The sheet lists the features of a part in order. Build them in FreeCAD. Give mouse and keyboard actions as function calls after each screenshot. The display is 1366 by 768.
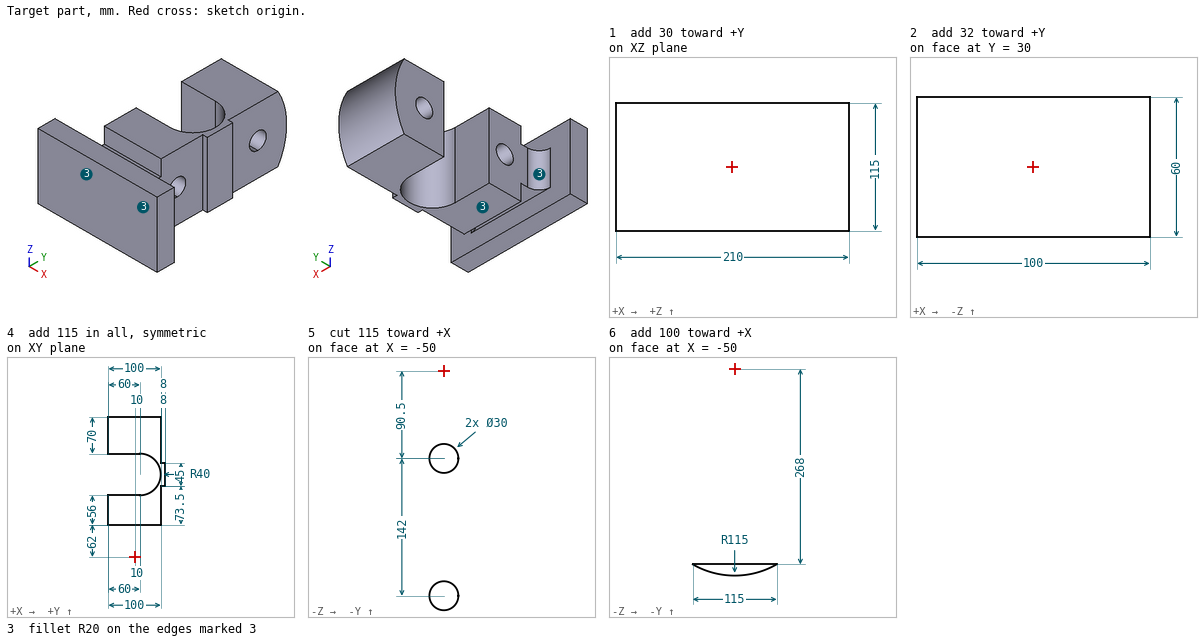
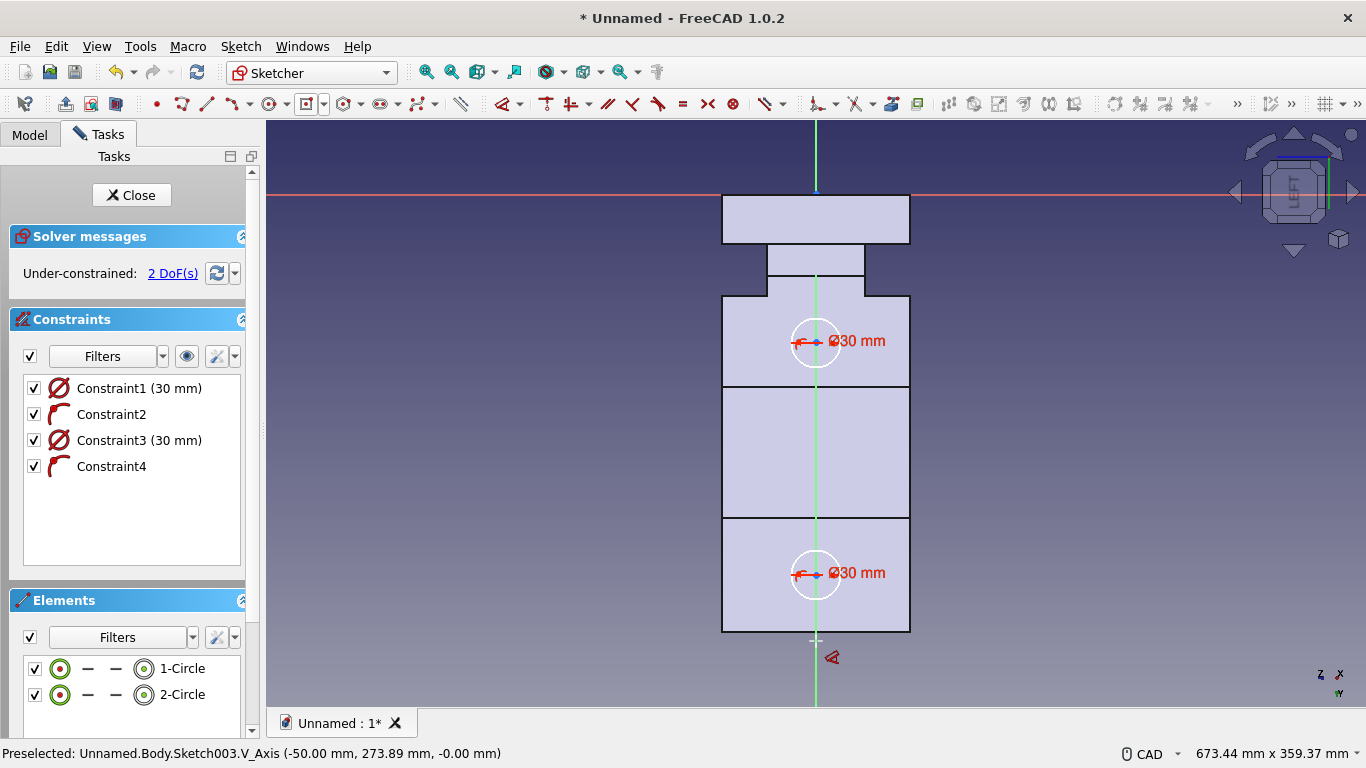
click(816, 343)
click(850, 269)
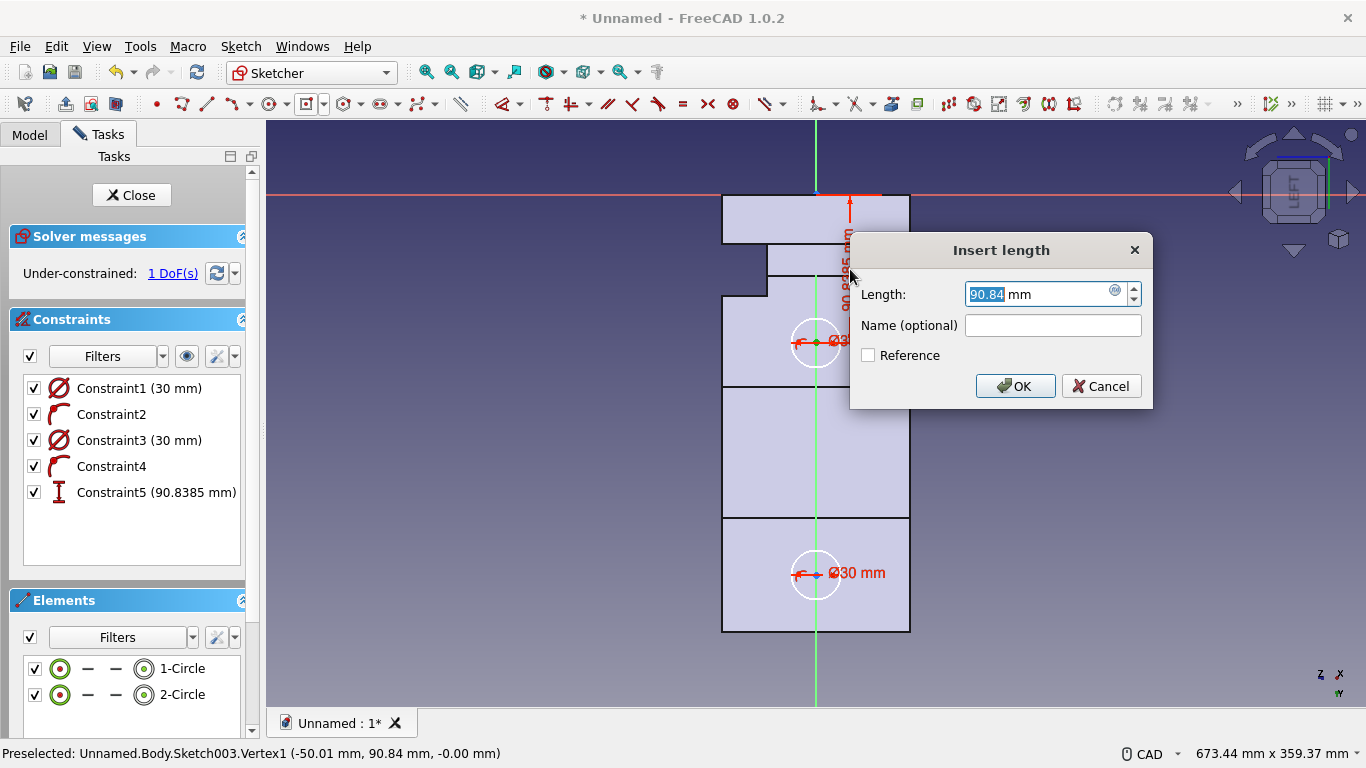
text(90.5)
key(Return)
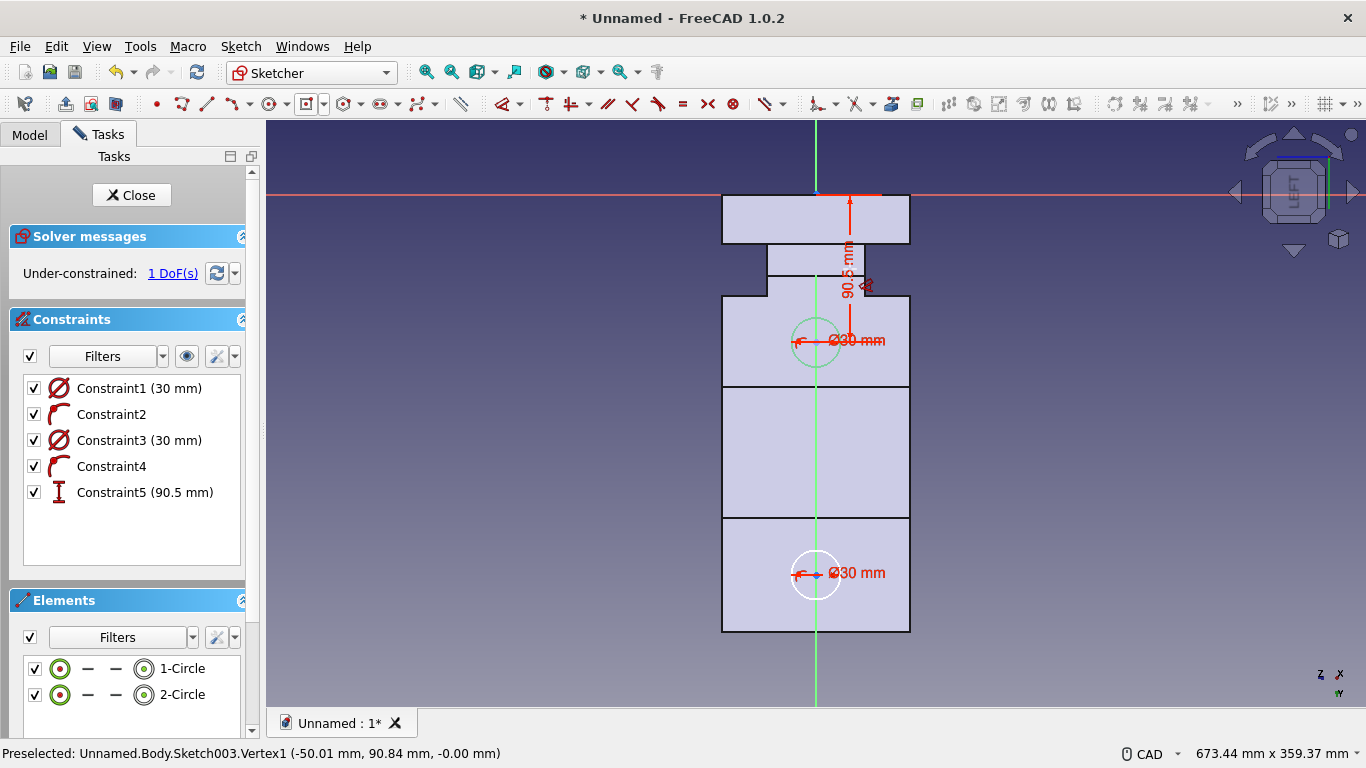
click(816, 342)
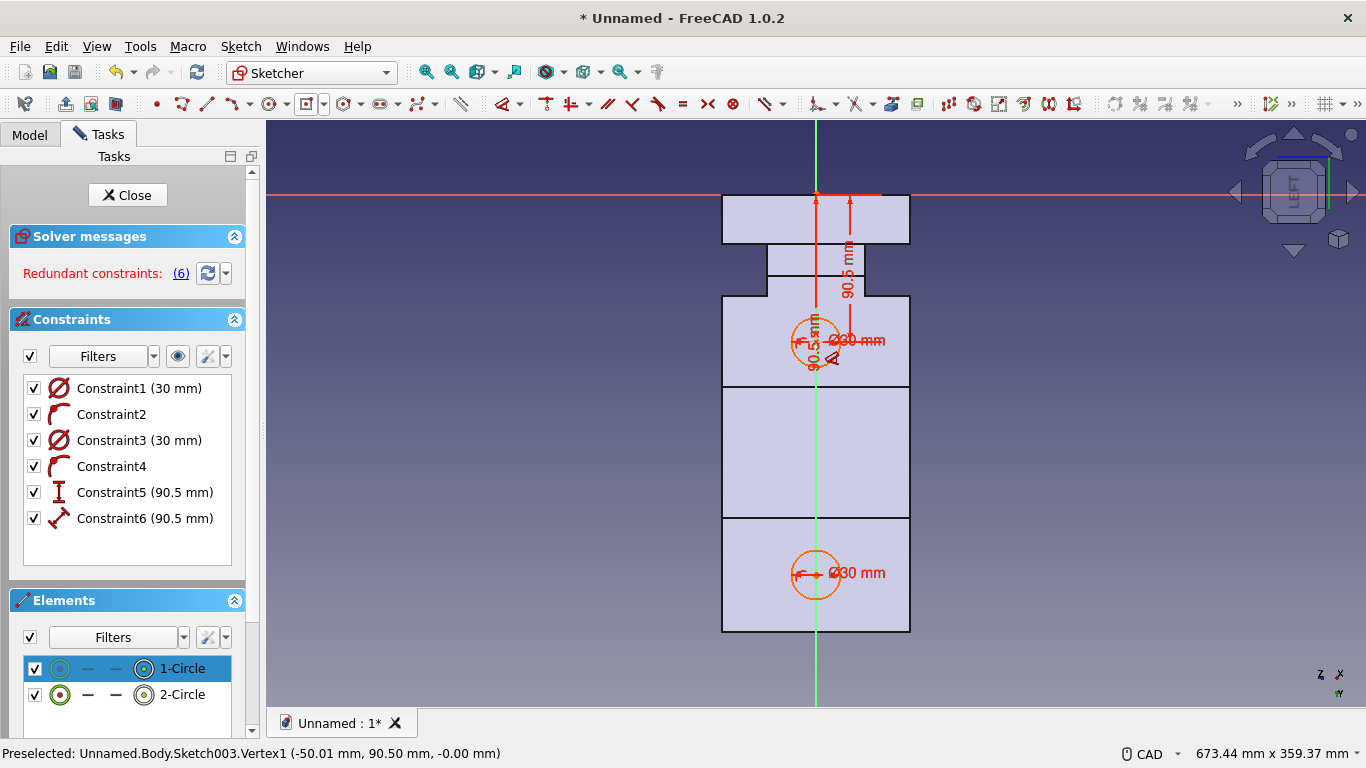
click(816, 575)
click(850, 459)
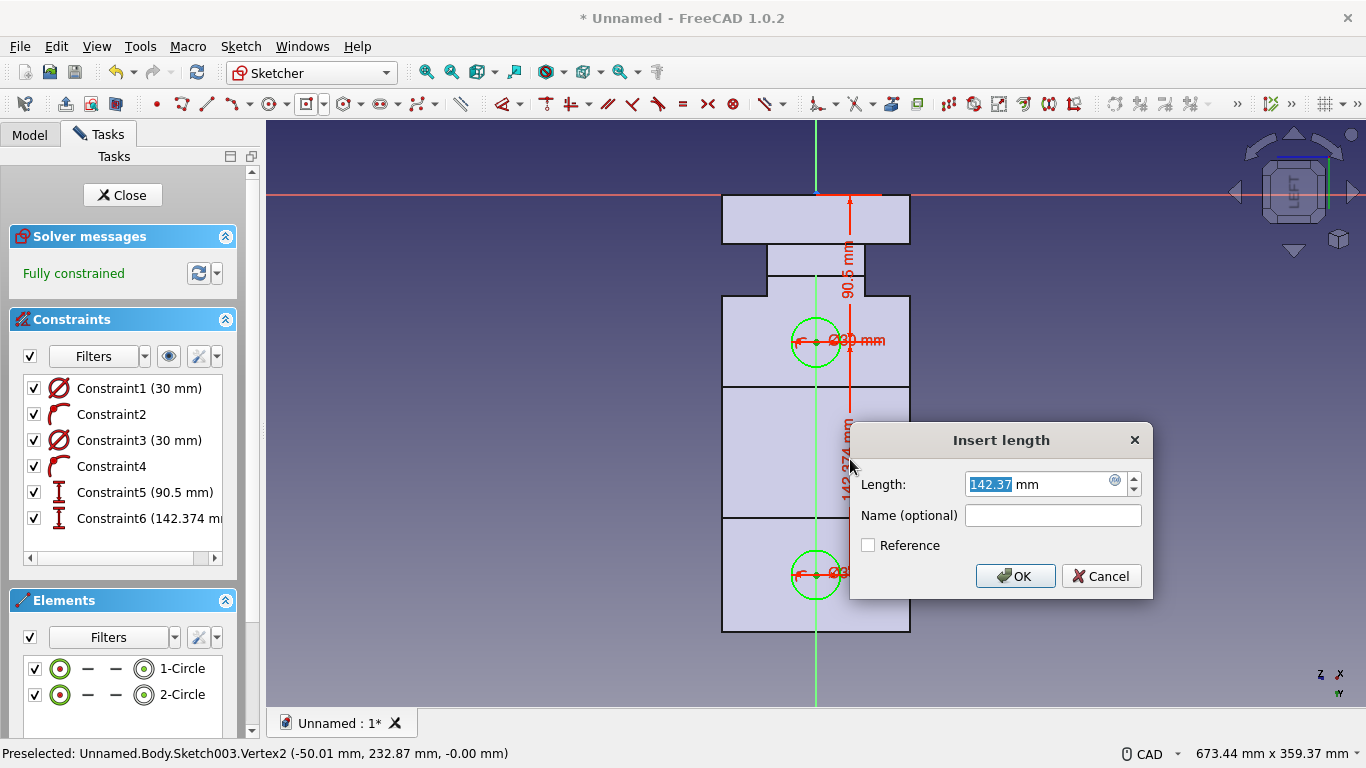
text(142)
key(Return)
key(Escape)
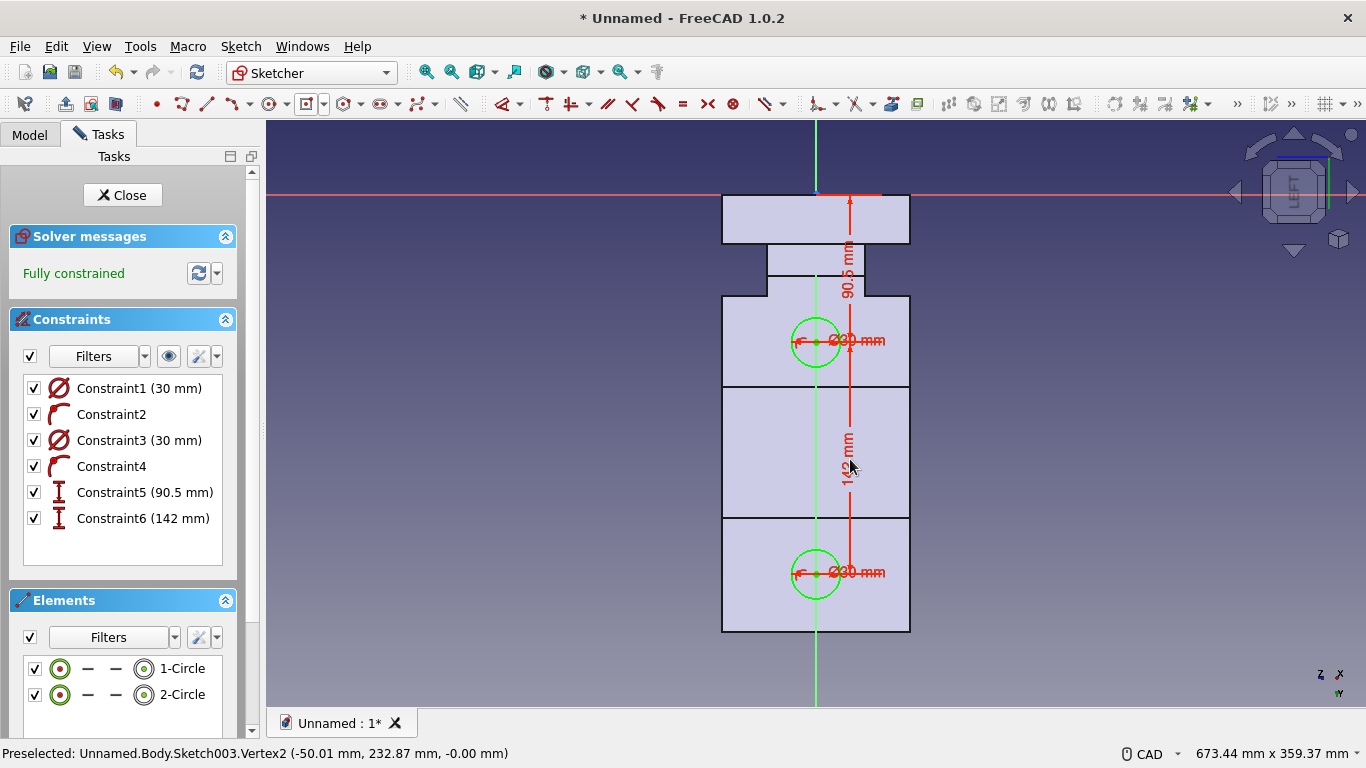
click(123, 195)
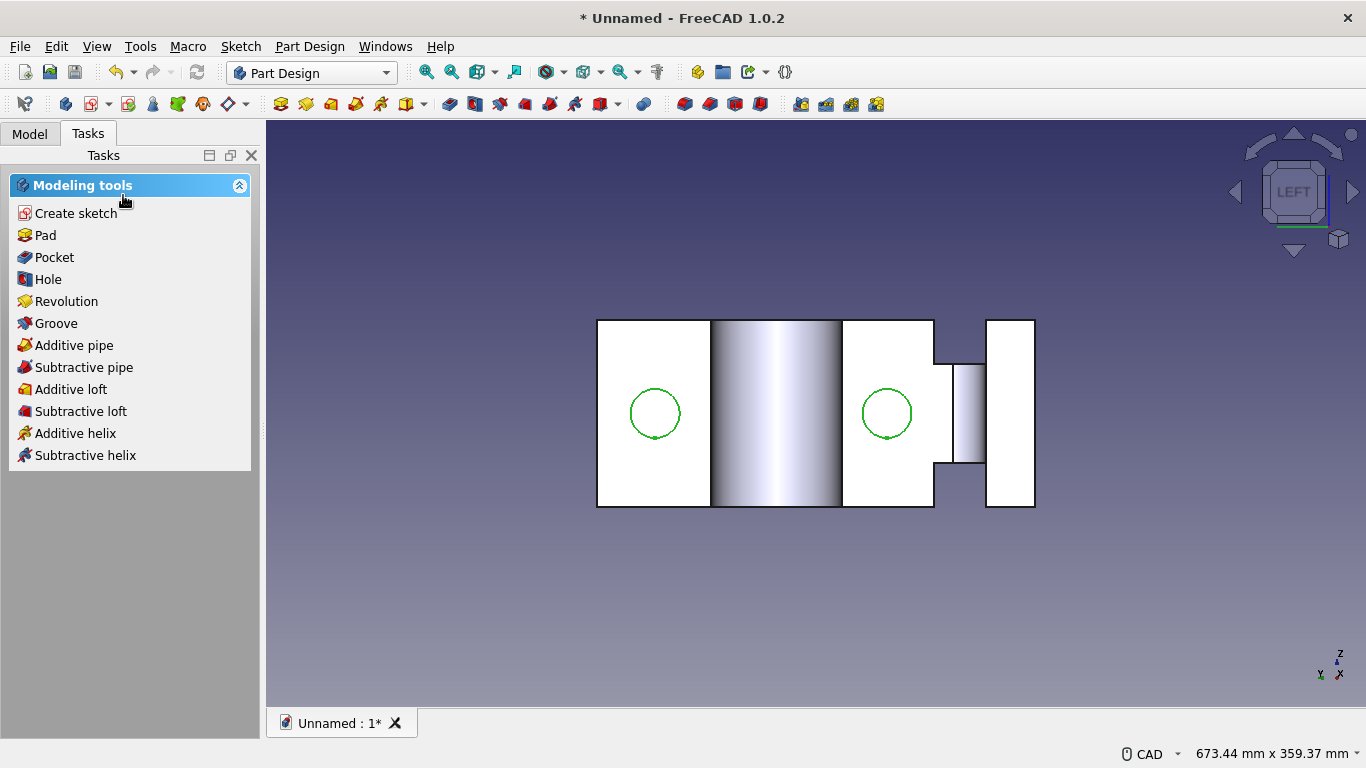
click(450, 104)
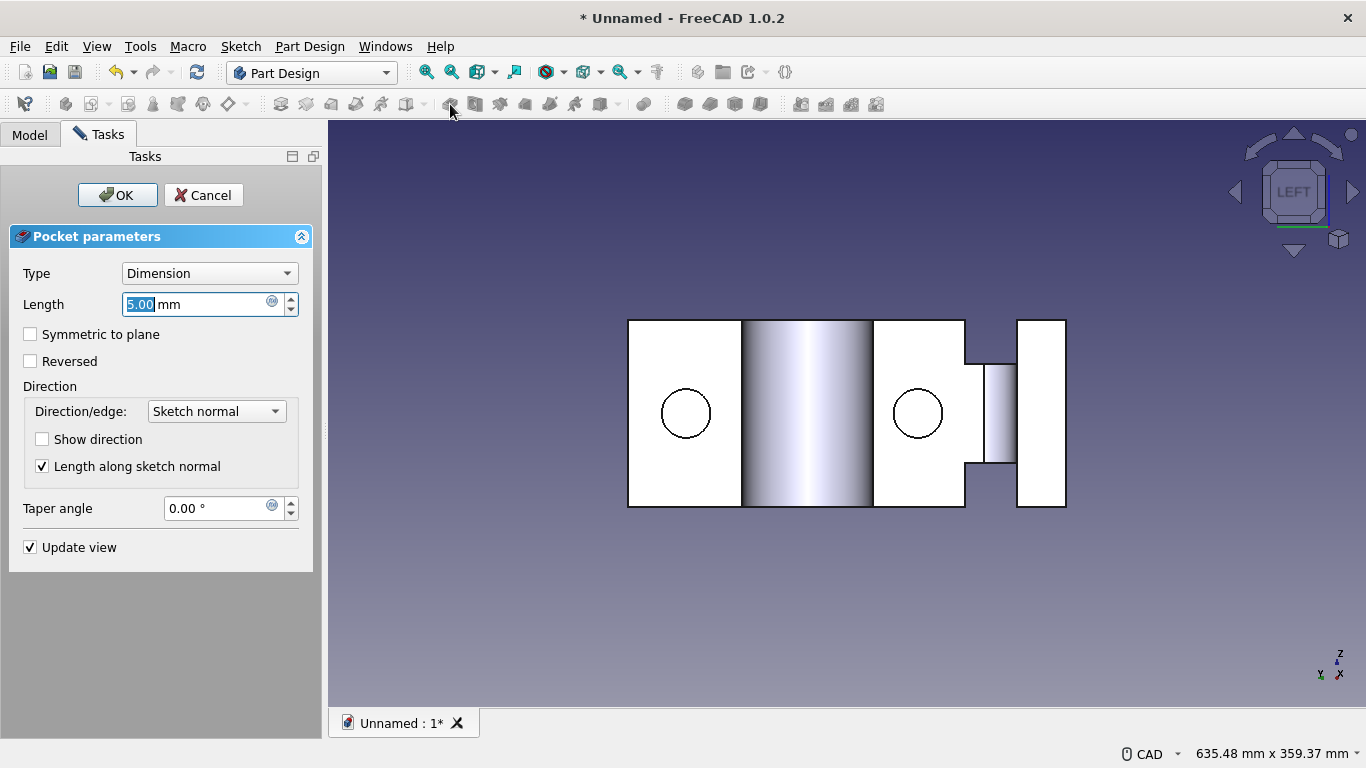
text(115)
key(Tab)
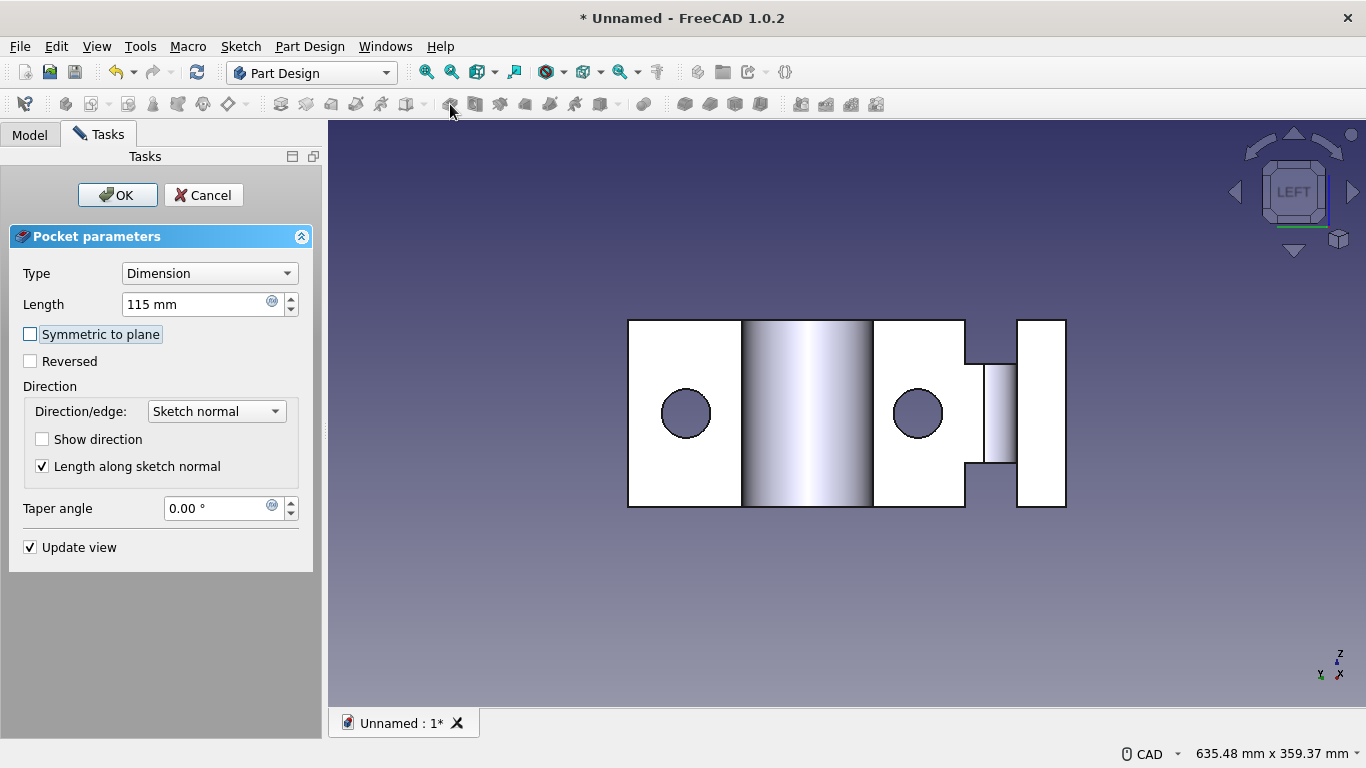
click(118, 195)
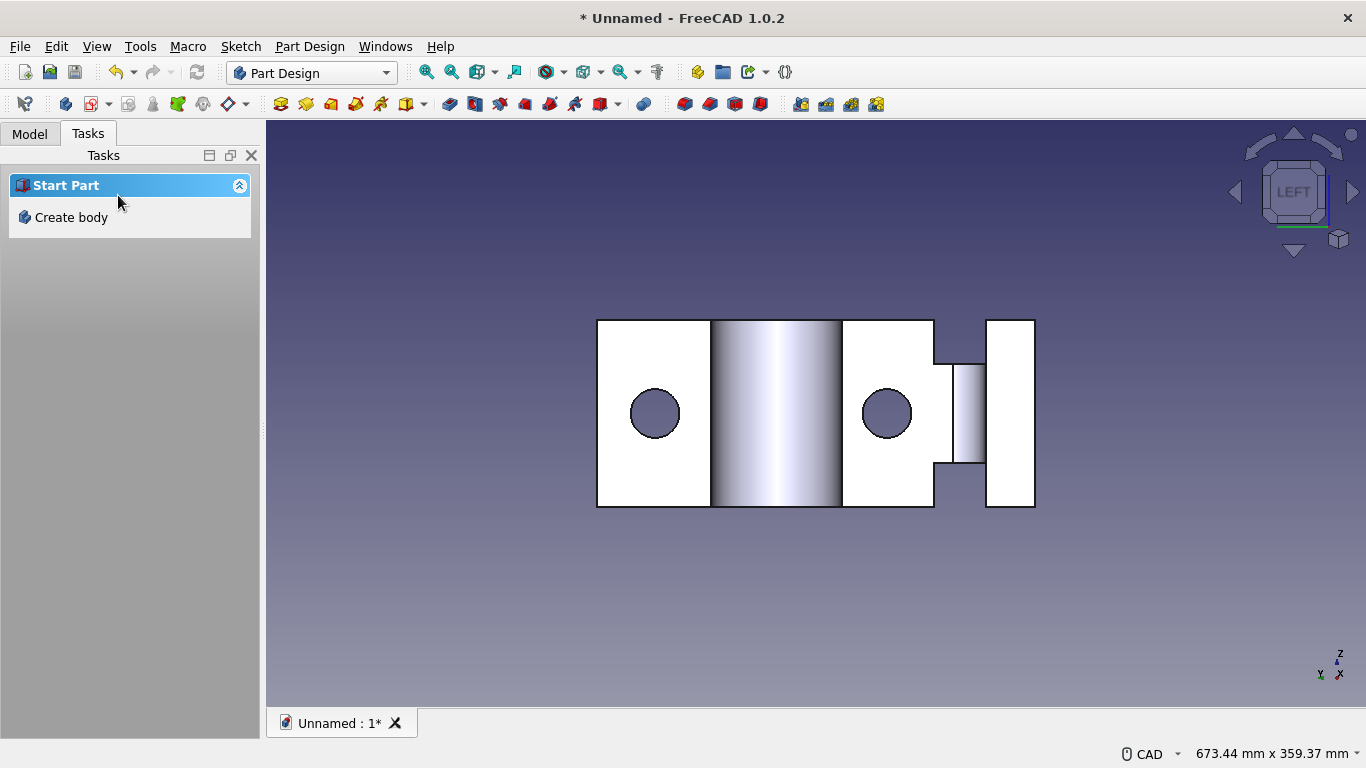
key(v)
key(f)